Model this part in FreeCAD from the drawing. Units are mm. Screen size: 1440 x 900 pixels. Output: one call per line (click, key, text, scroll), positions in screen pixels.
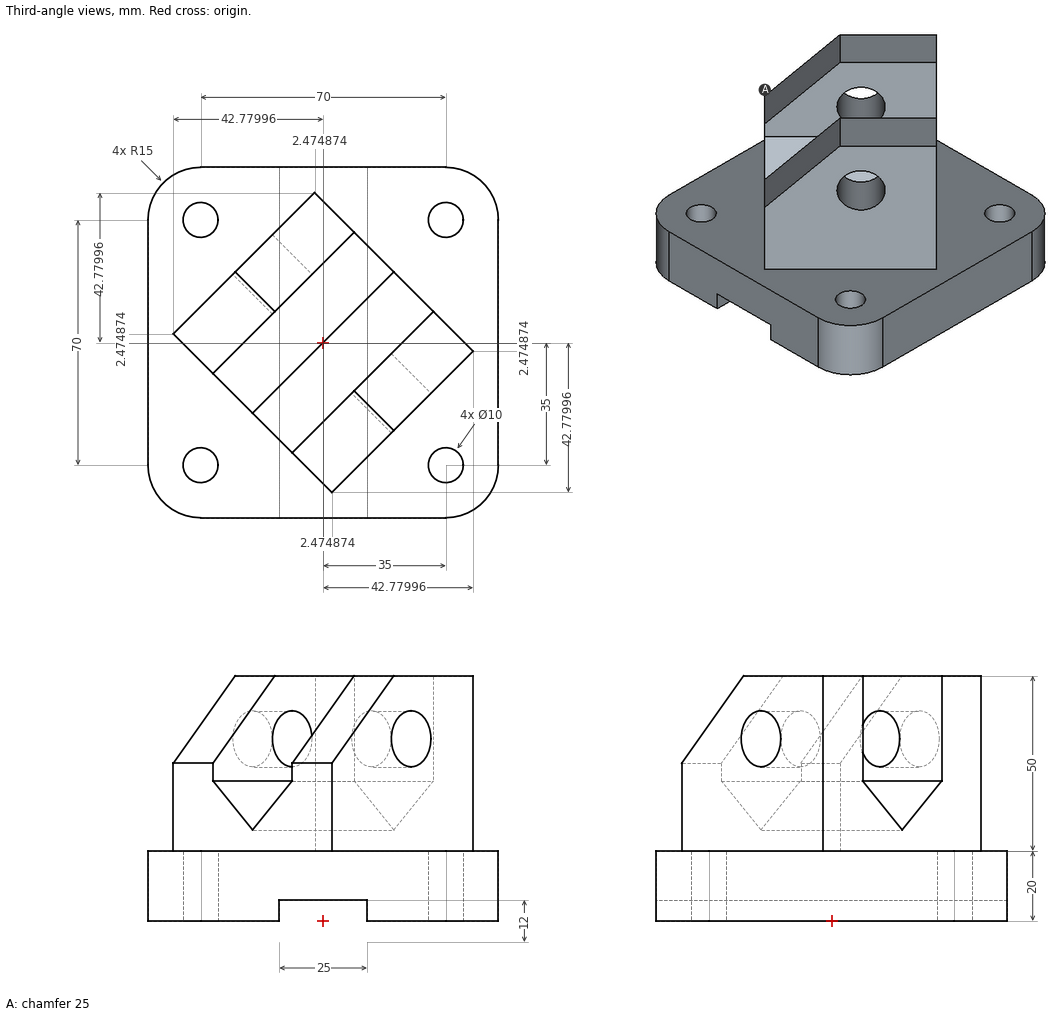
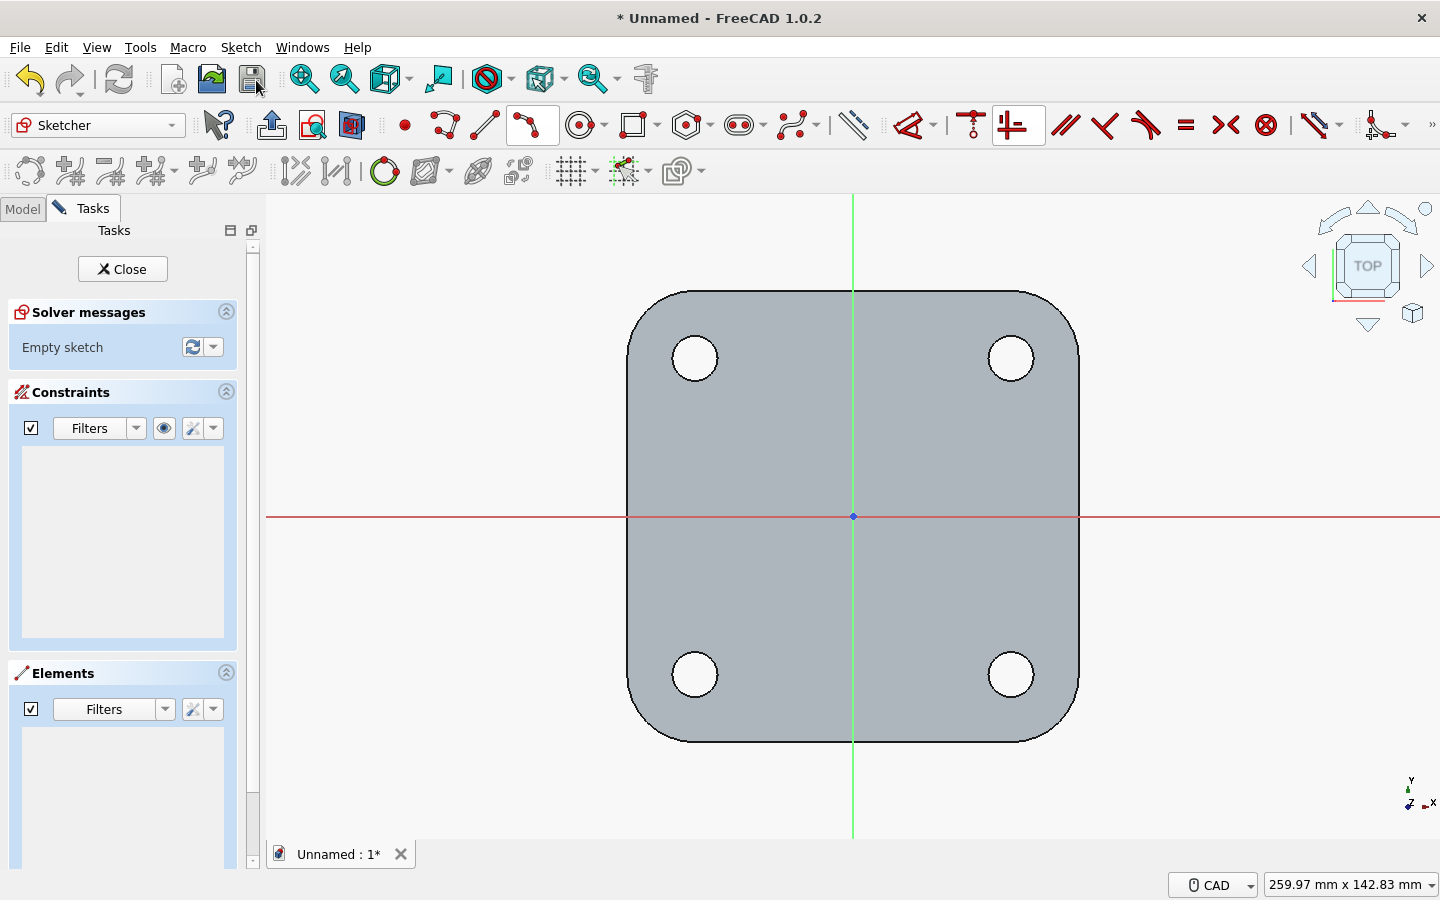
scroll(842, 323, up, 2)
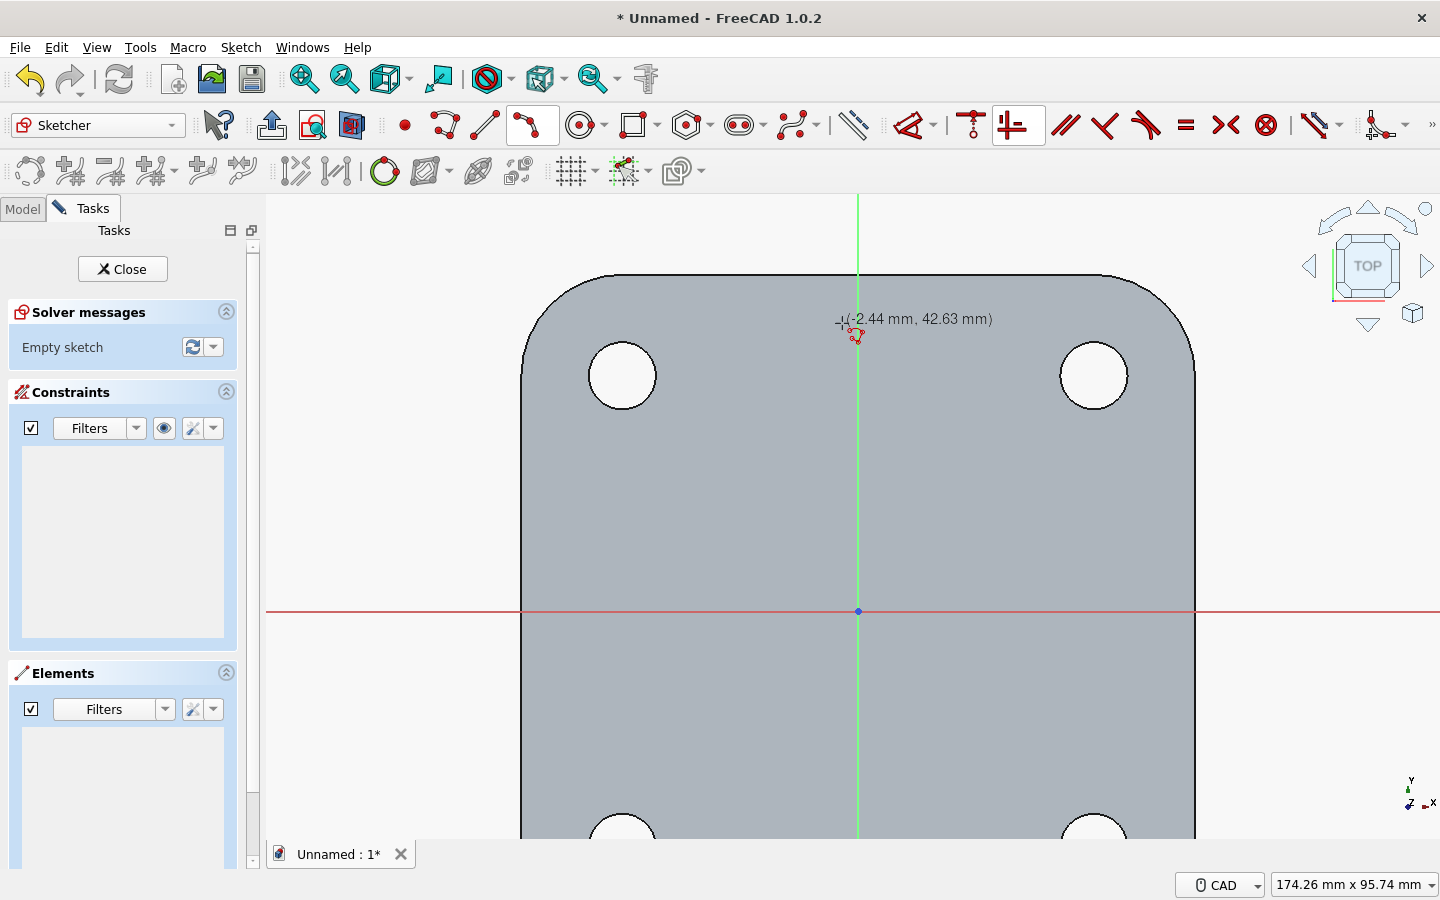
click(841, 323)
click(570, 595)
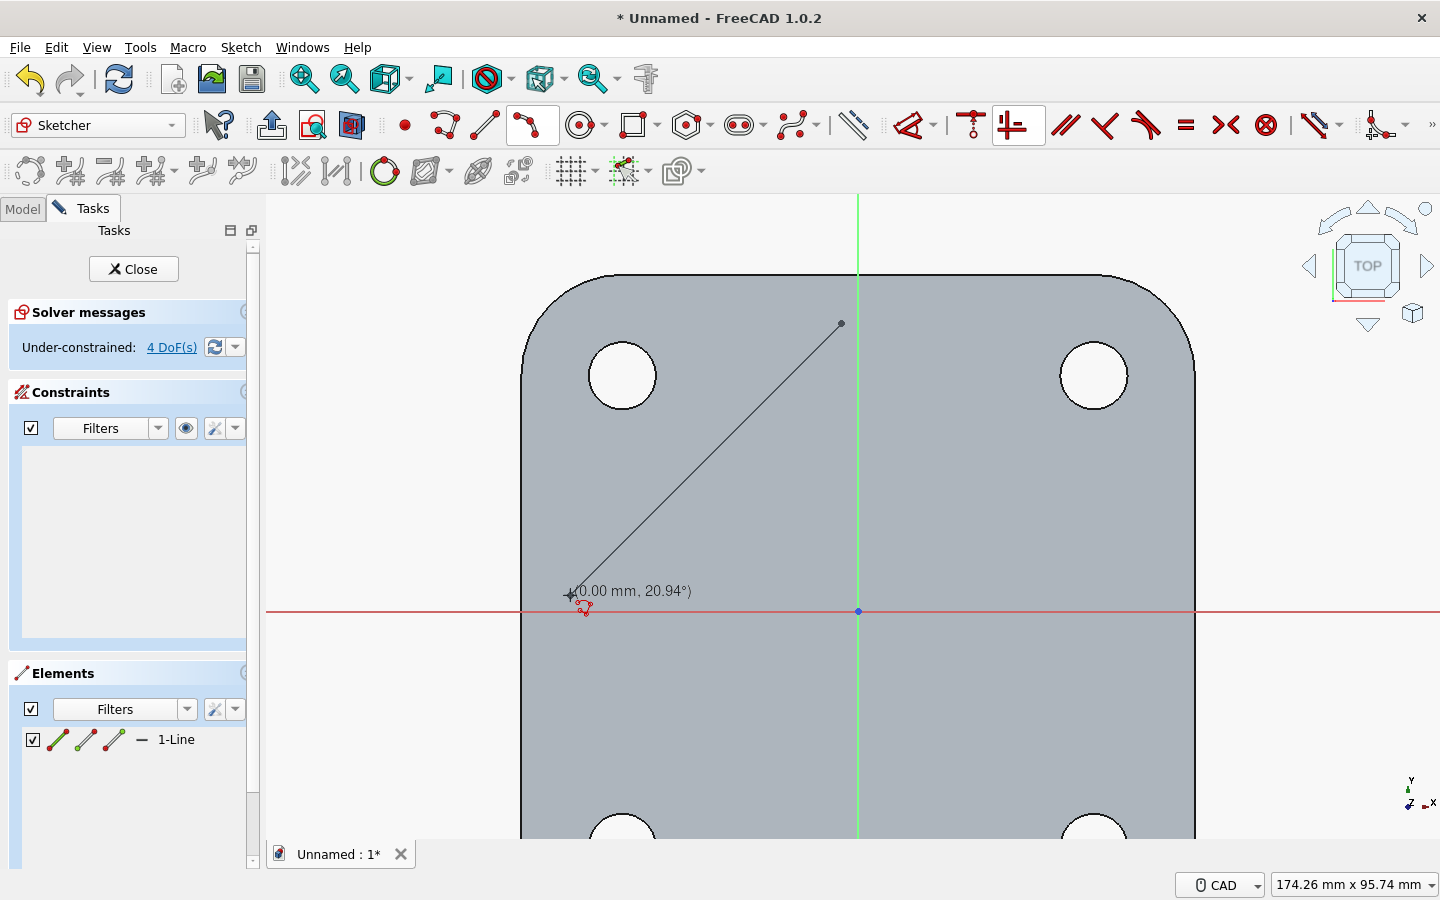
scroll(635, 323, down, 2)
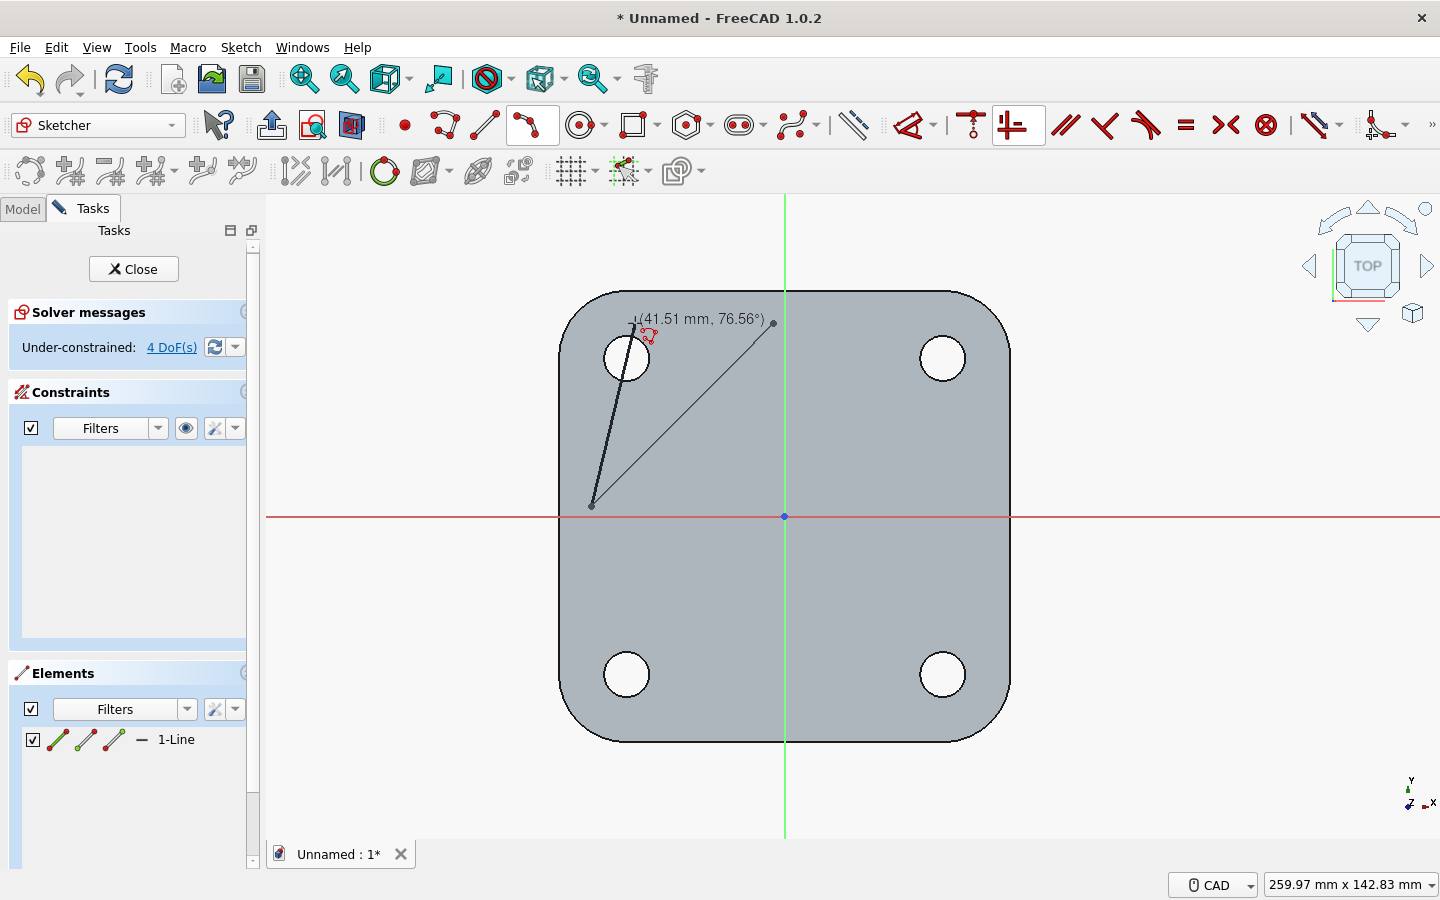
scroll(796, 710, up, 2)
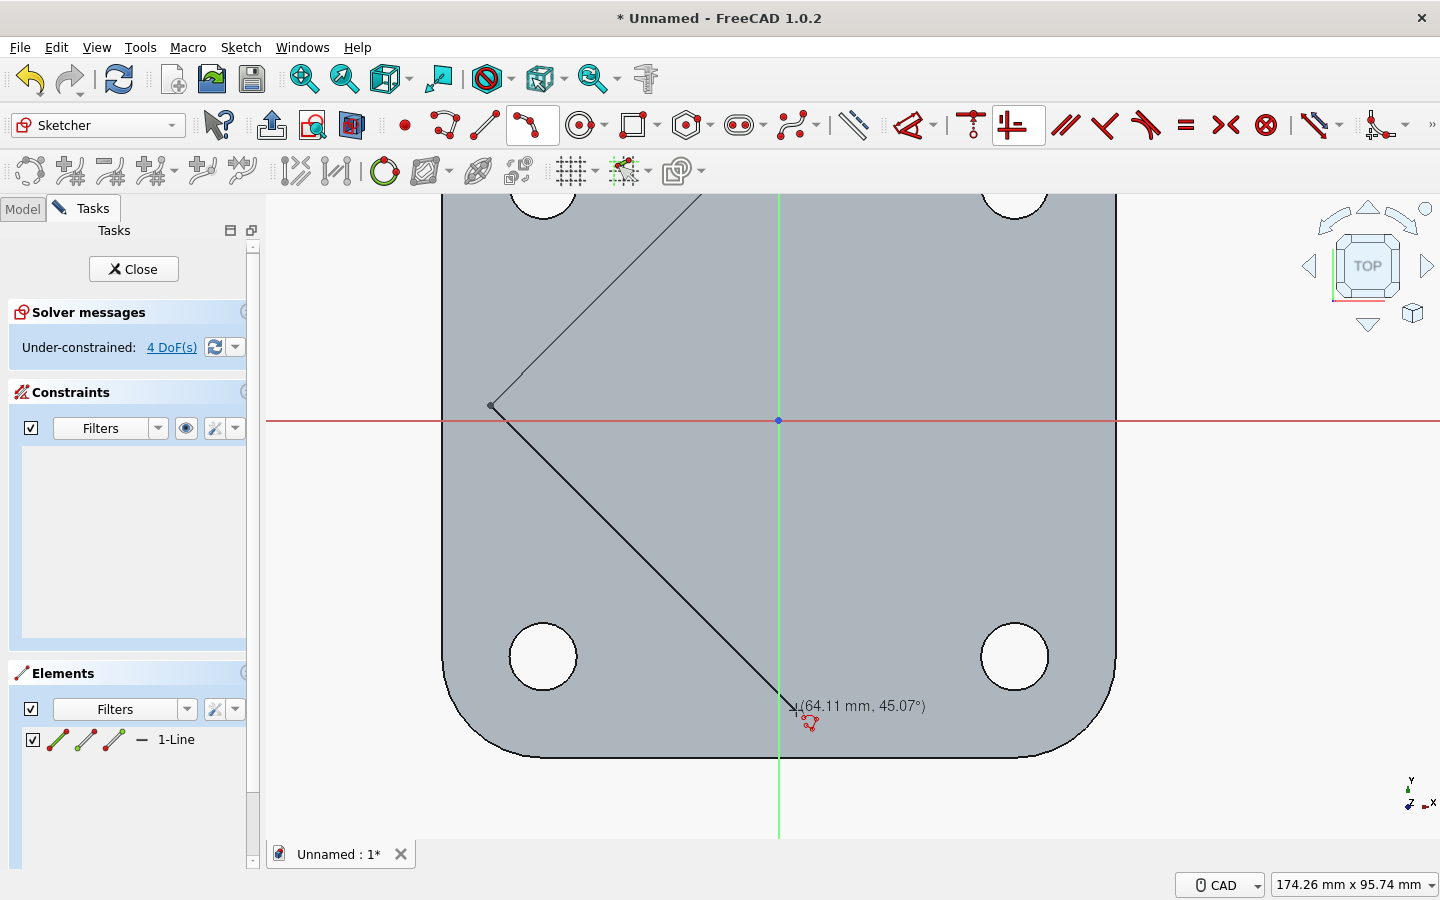
click(796, 709)
click(1067, 438)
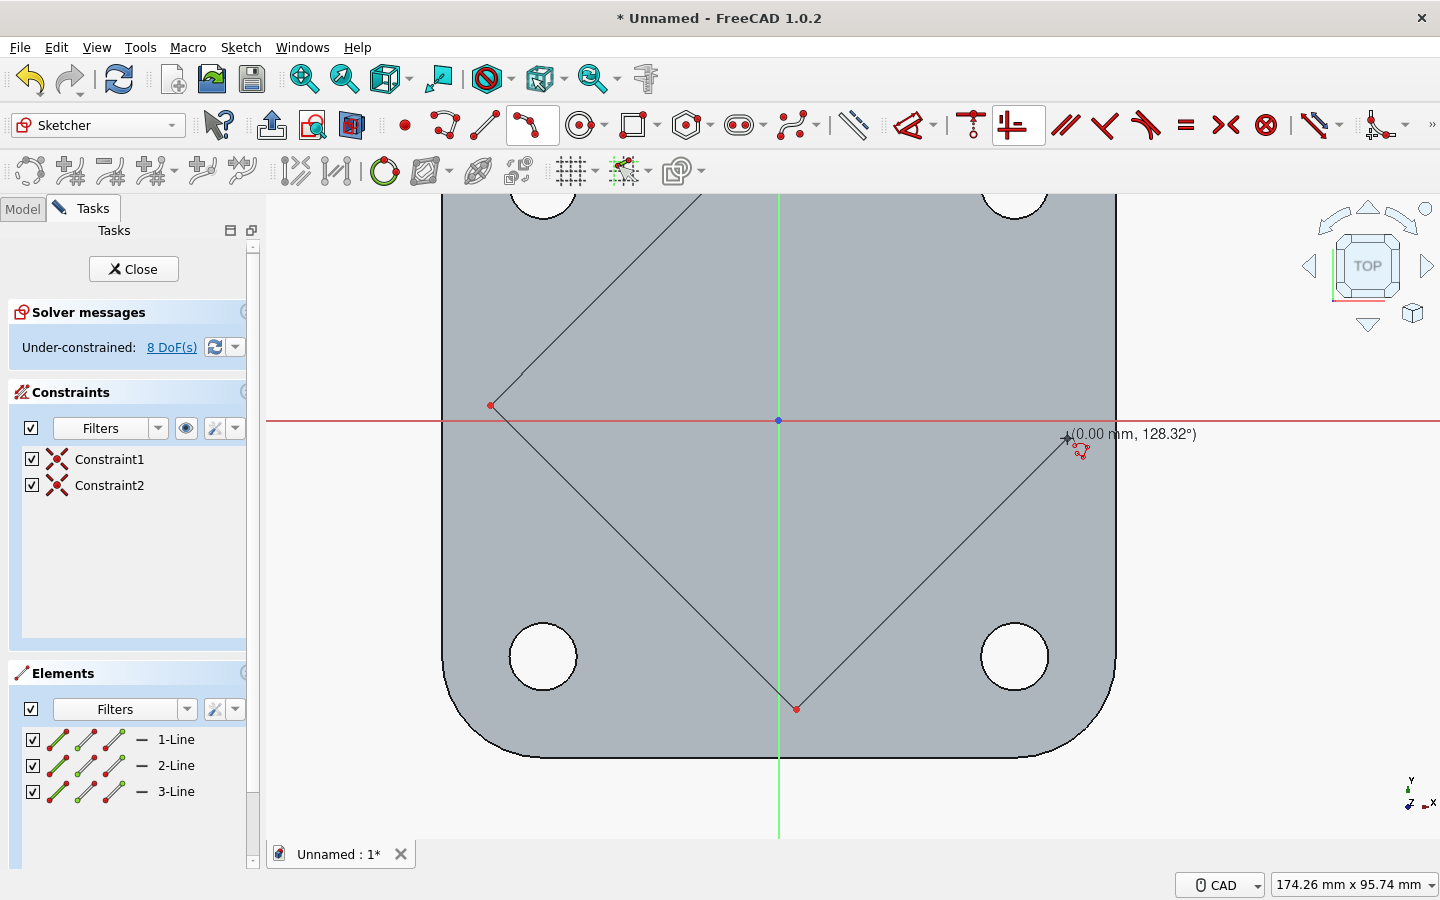
scroll(796, 711, down, 2)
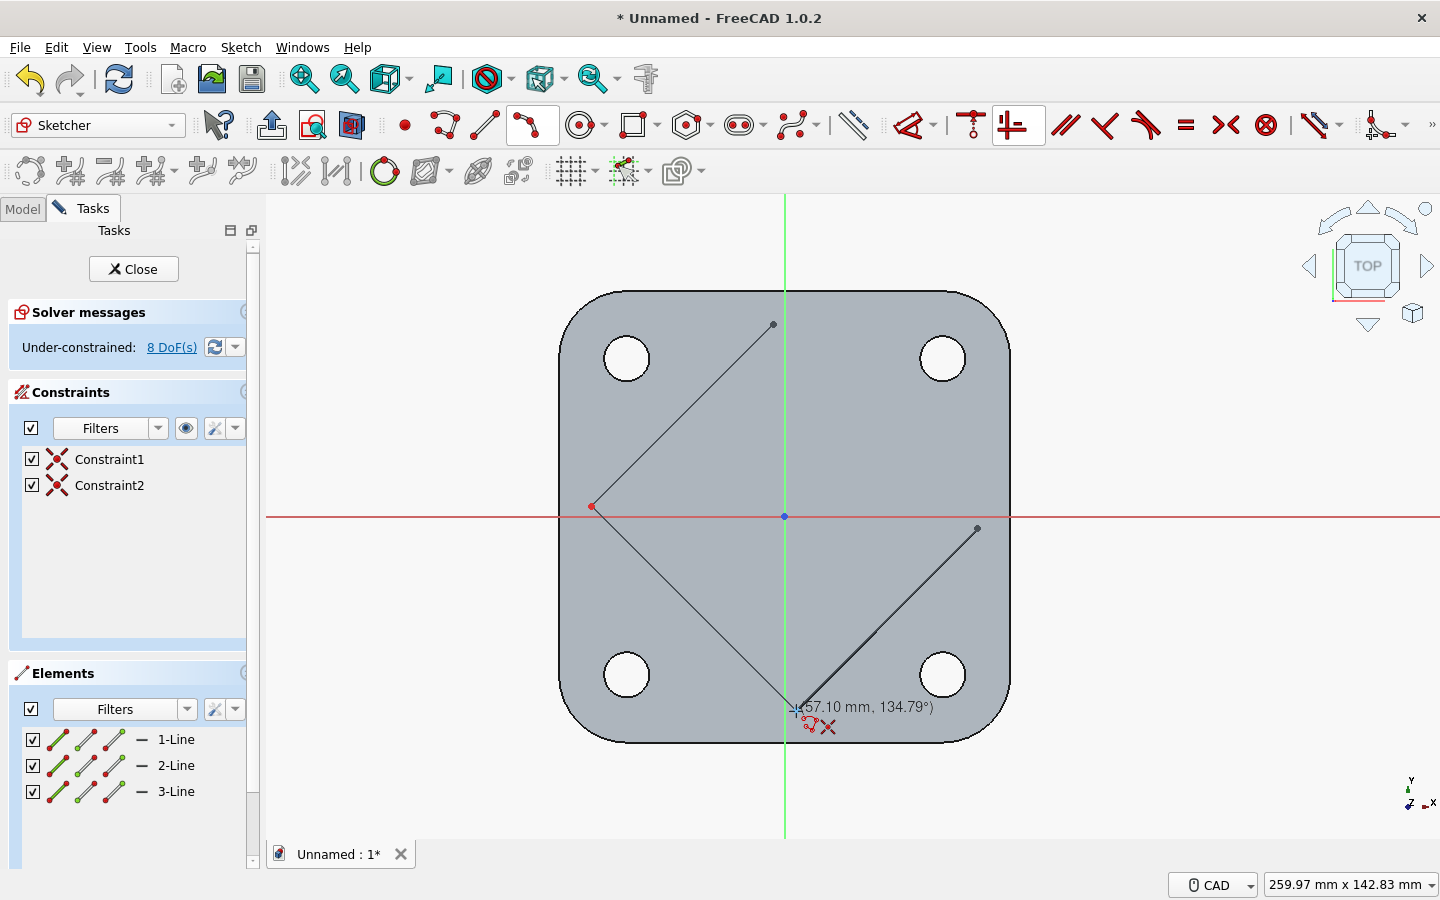
scroll(774, 324, up, 2)